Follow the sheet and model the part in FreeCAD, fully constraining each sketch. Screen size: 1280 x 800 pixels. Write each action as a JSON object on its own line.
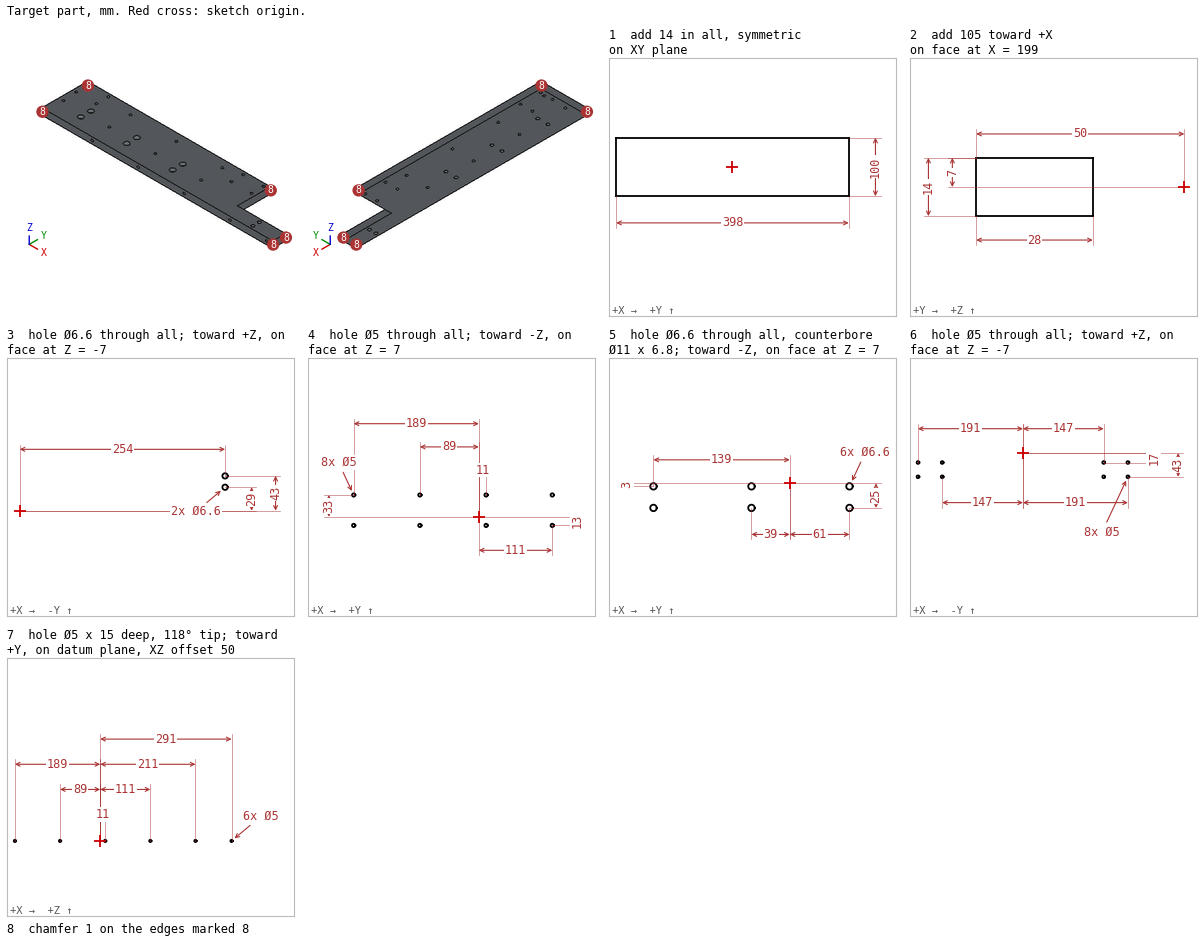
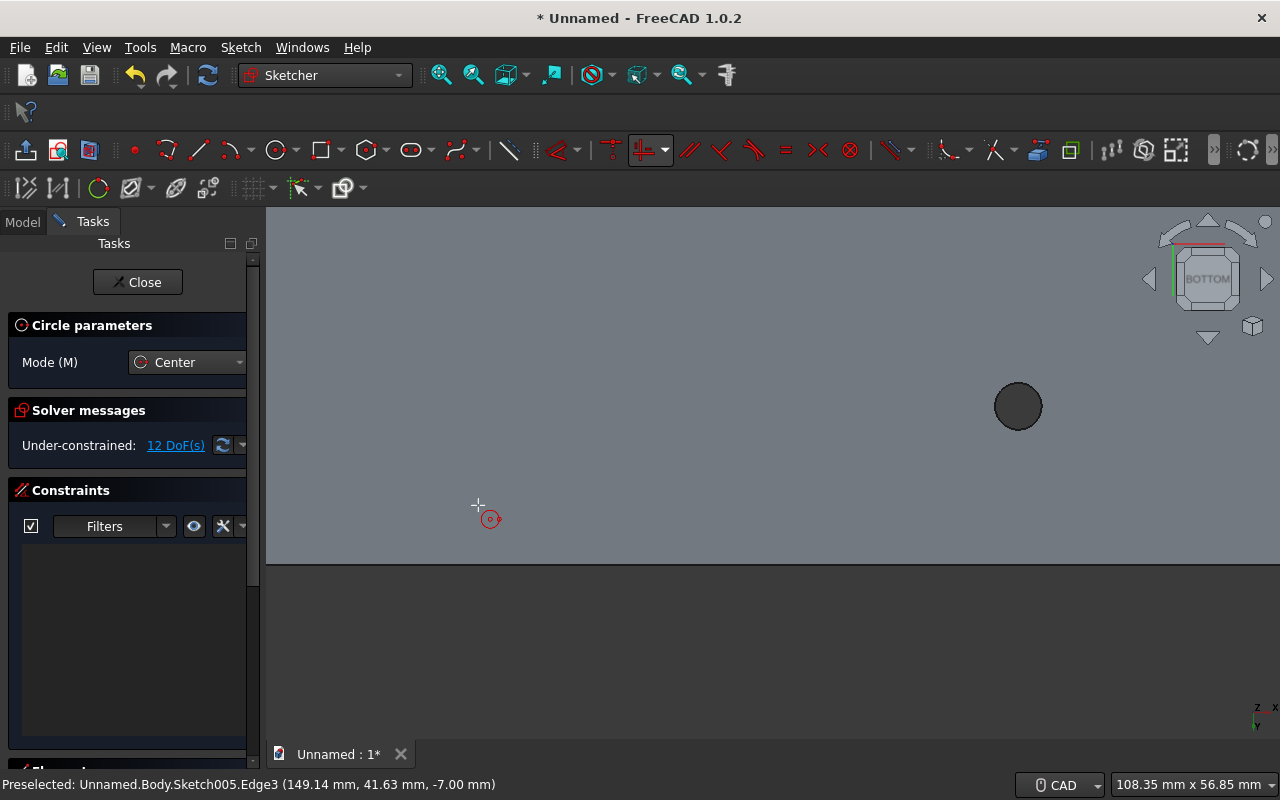
{"action": "scroll", "coordinate": [477, 505], "scroll_direction": "down", "scroll_amount": 9}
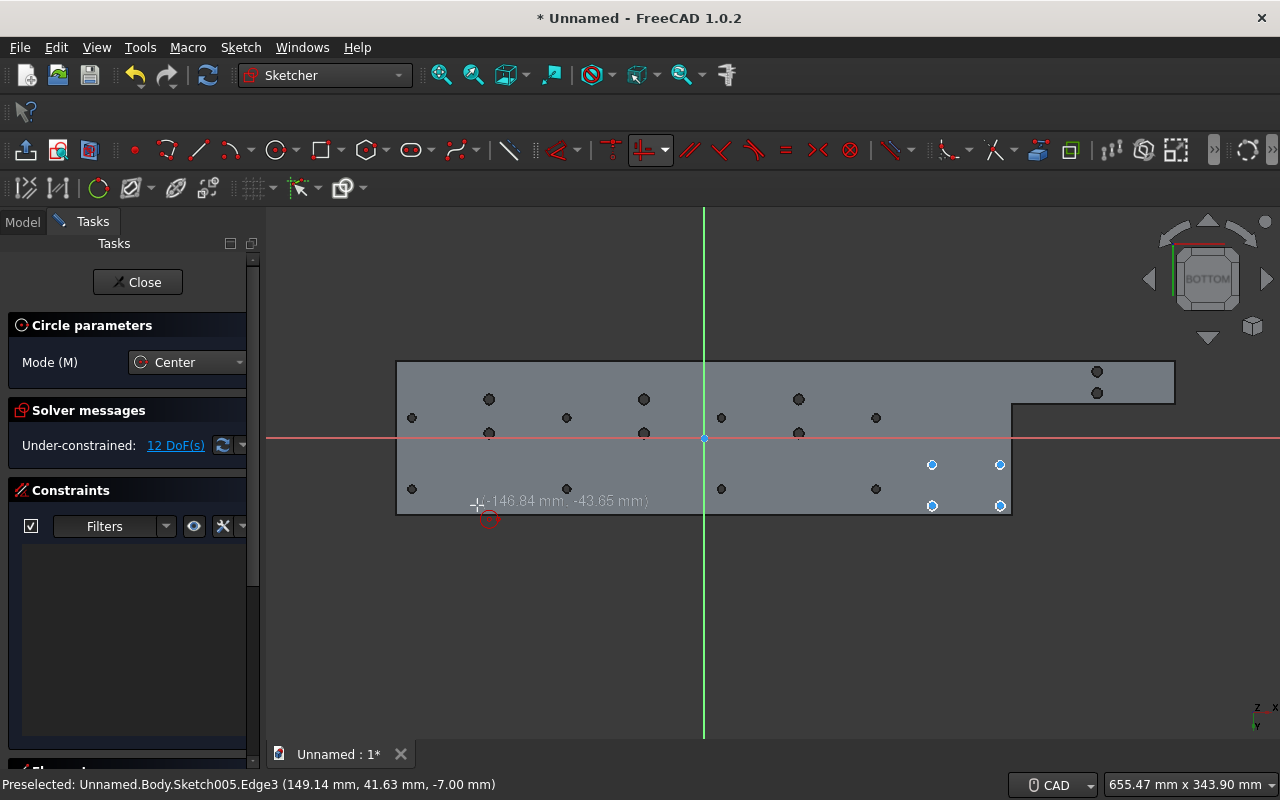
{"action": "left_click", "coordinate": [477, 505]}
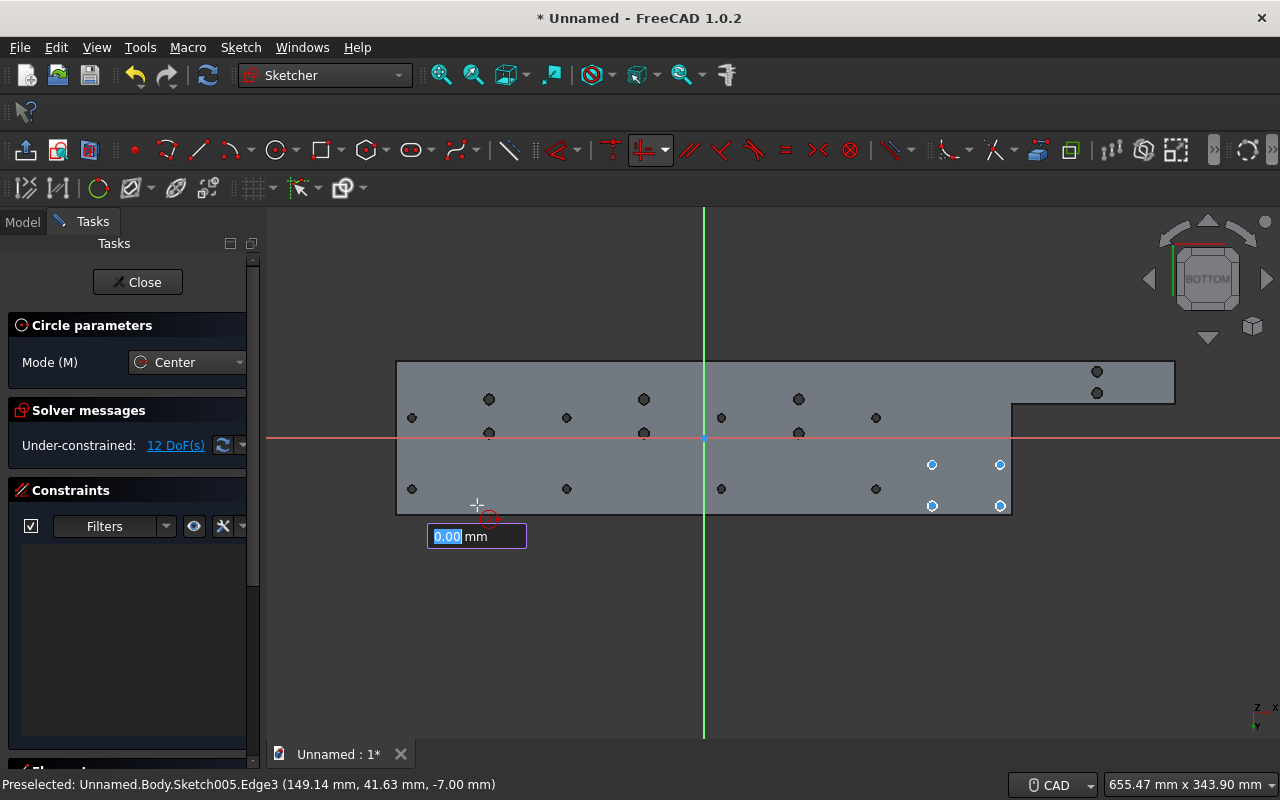
{"action": "scroll", "coordinate": [480, 502], "scroll_direction": "up", "scroll_amount": 8}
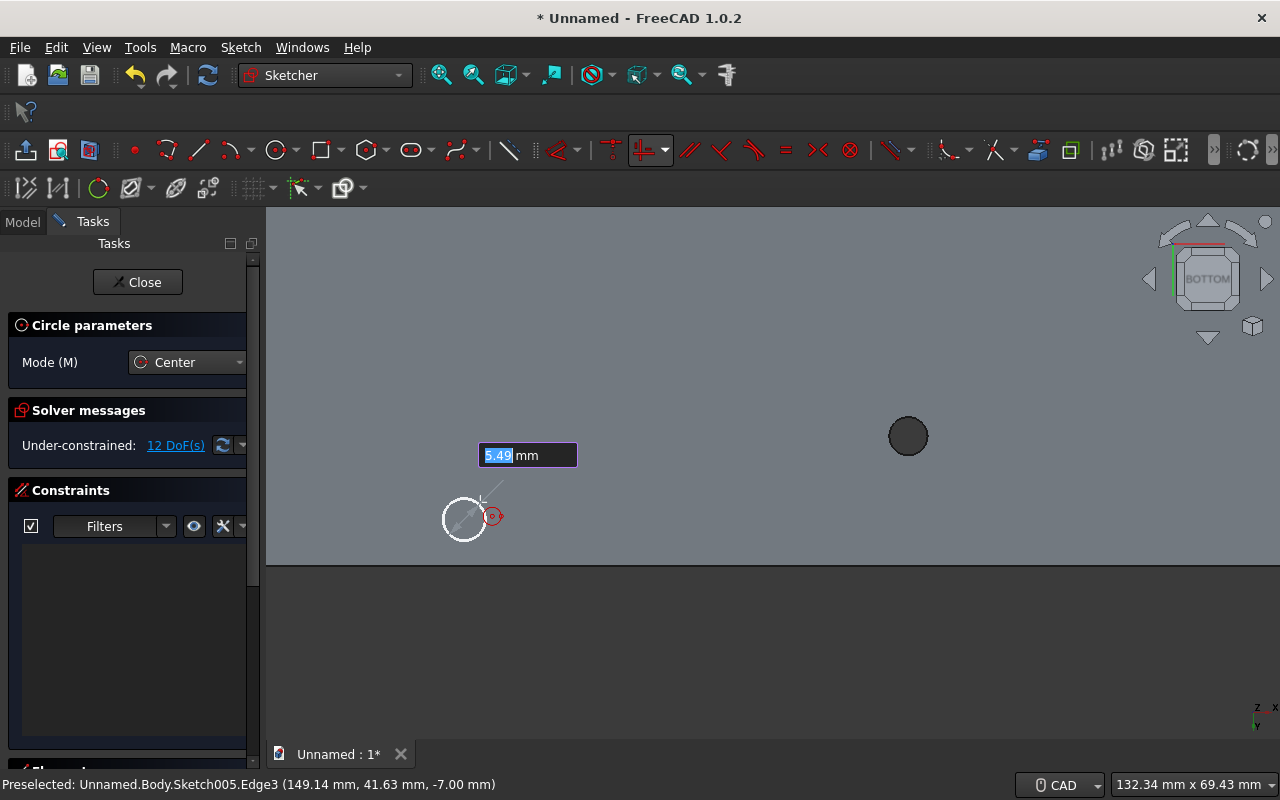
{"action": "left_click", "coordinate": [478, 499]}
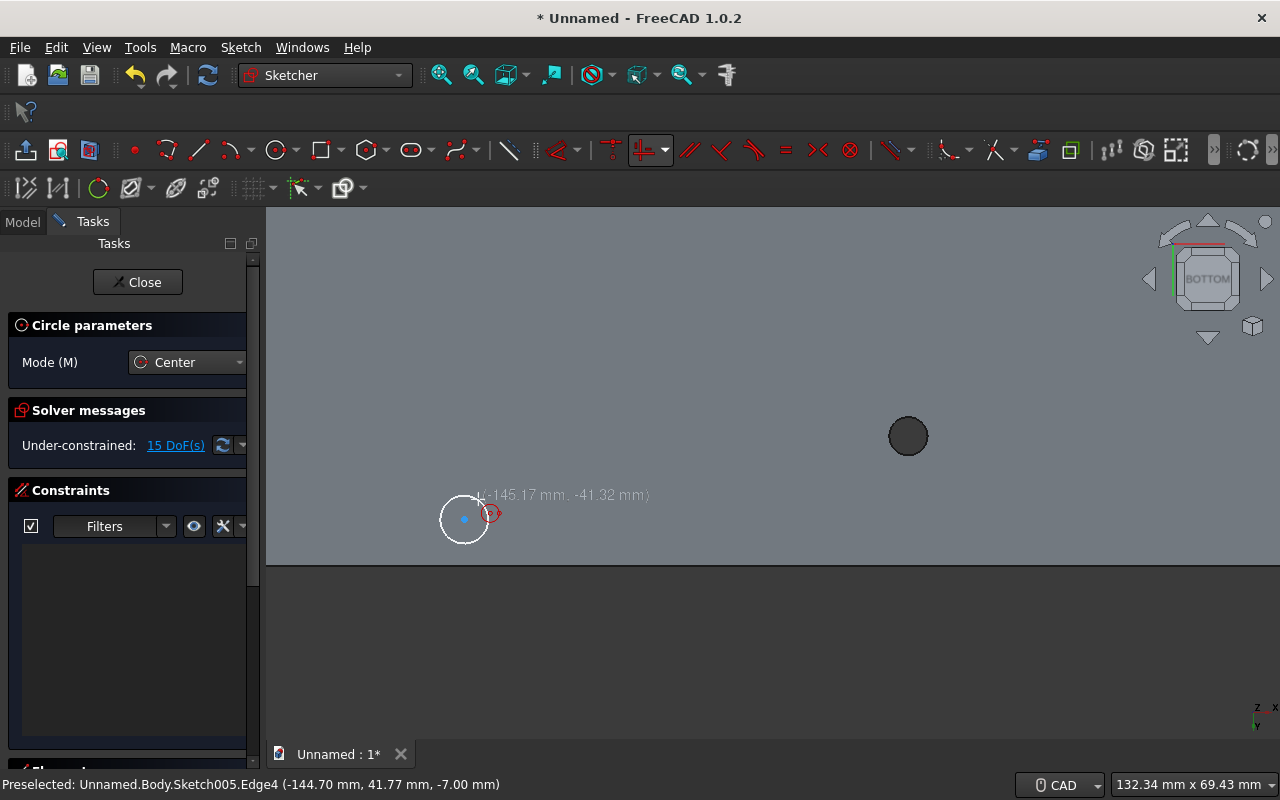
{"action": "scroll", "coordinate": [480, 502], "scroll_direction": "down", "scroll_amount": 8}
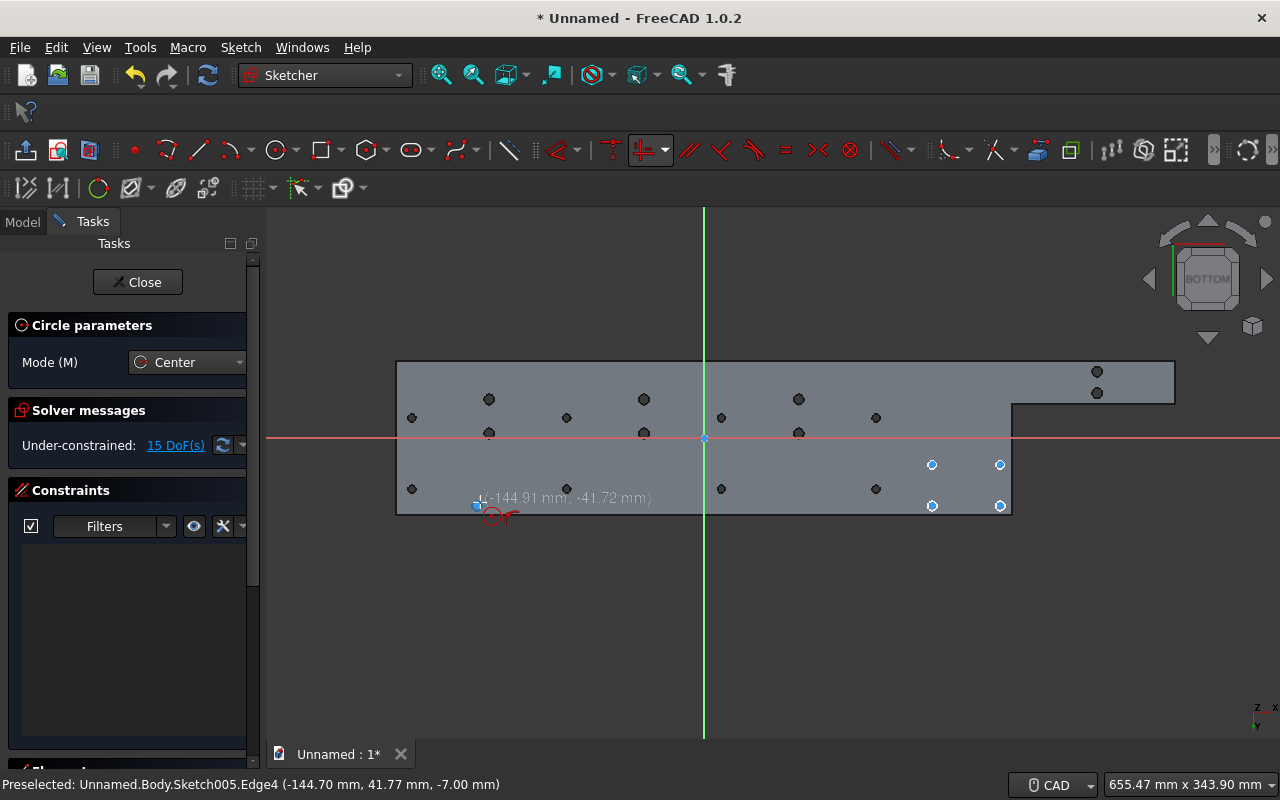
{"action": "scroll", "coordinate": [409, 464], "scroll_direction": "up", "scroll_amount": 9}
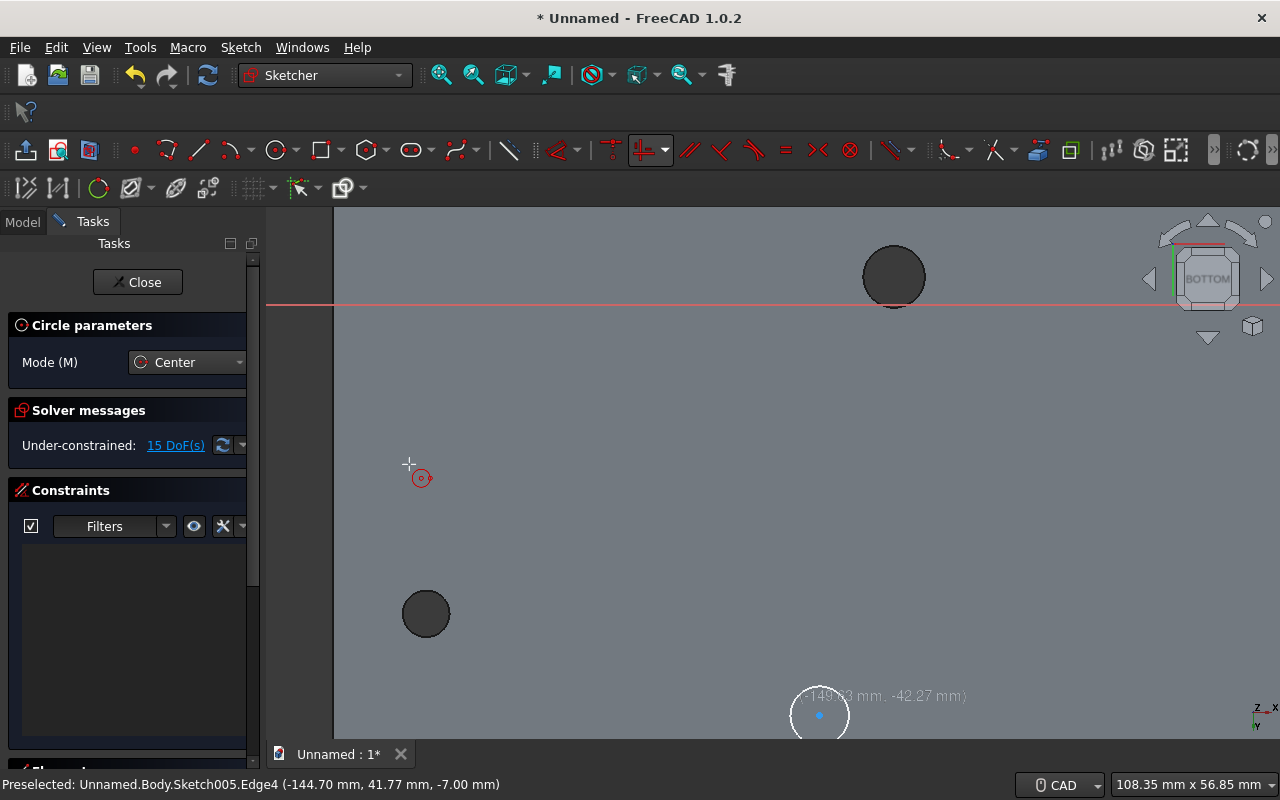
{"action": "scroll", "coordinate": [409, 464], "scroll_direction": "down", "scroll_amount": 9}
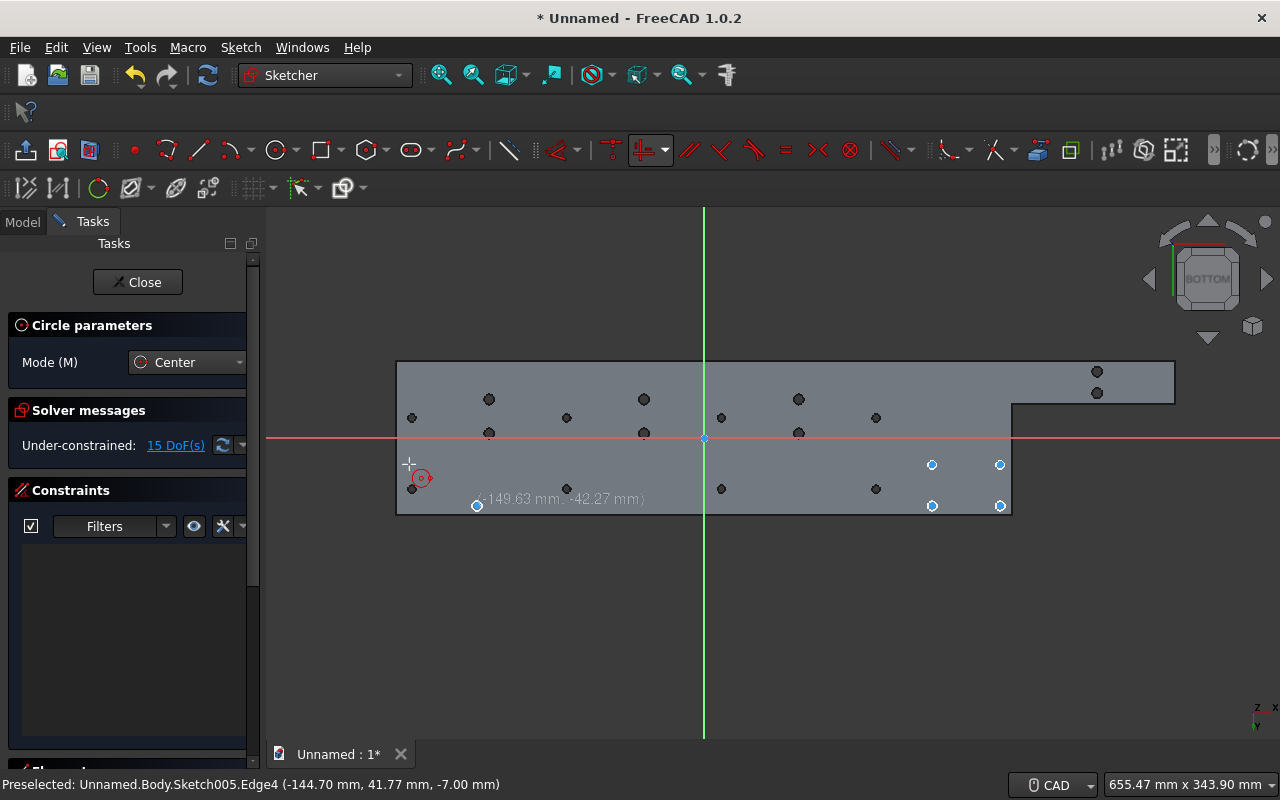
{"action": "left_click", "coordinate": [409, 464]}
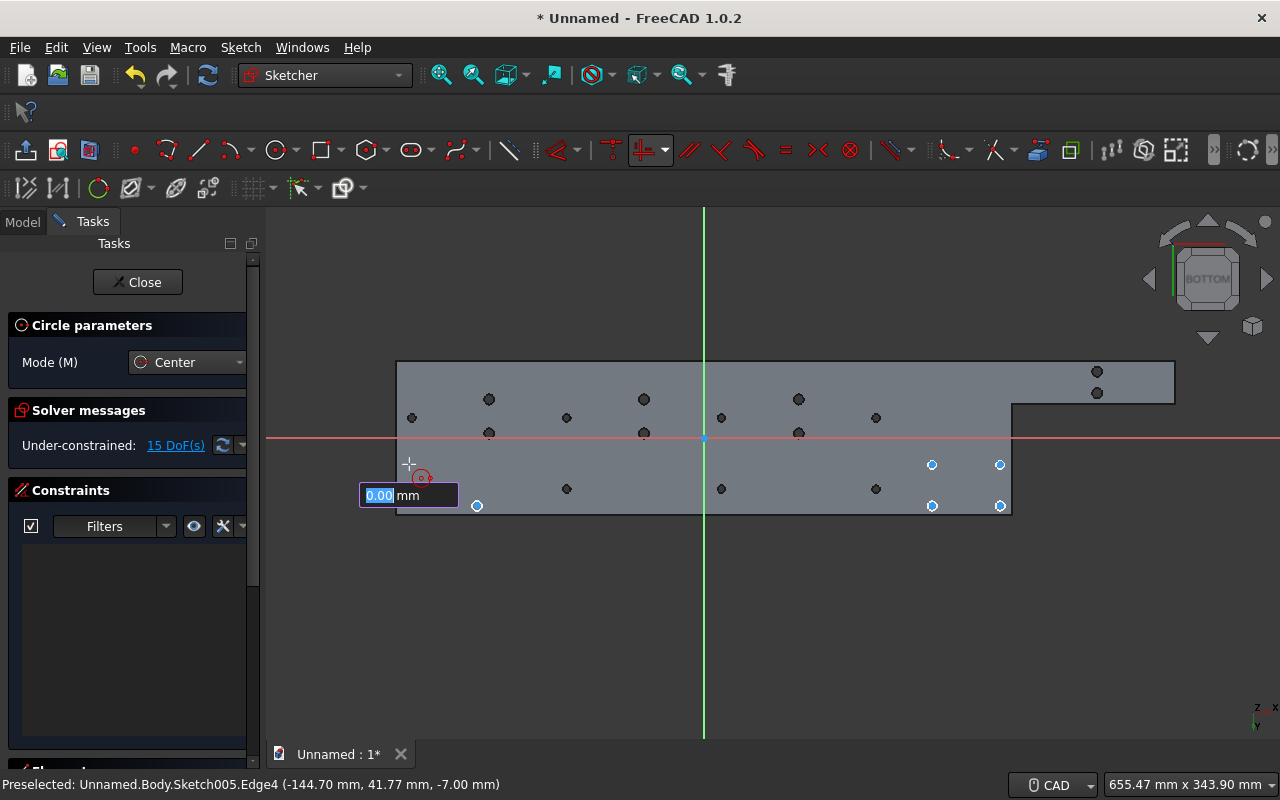
{"action": "scroll", "coordinate": [412, 462], "scroll_direction": "up", "scroll_amount": 8}